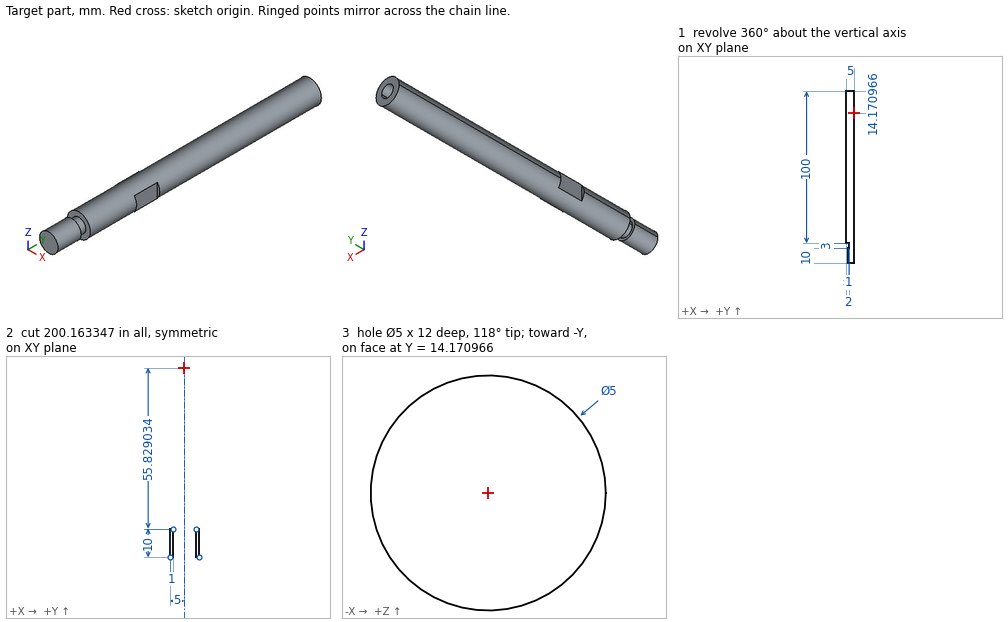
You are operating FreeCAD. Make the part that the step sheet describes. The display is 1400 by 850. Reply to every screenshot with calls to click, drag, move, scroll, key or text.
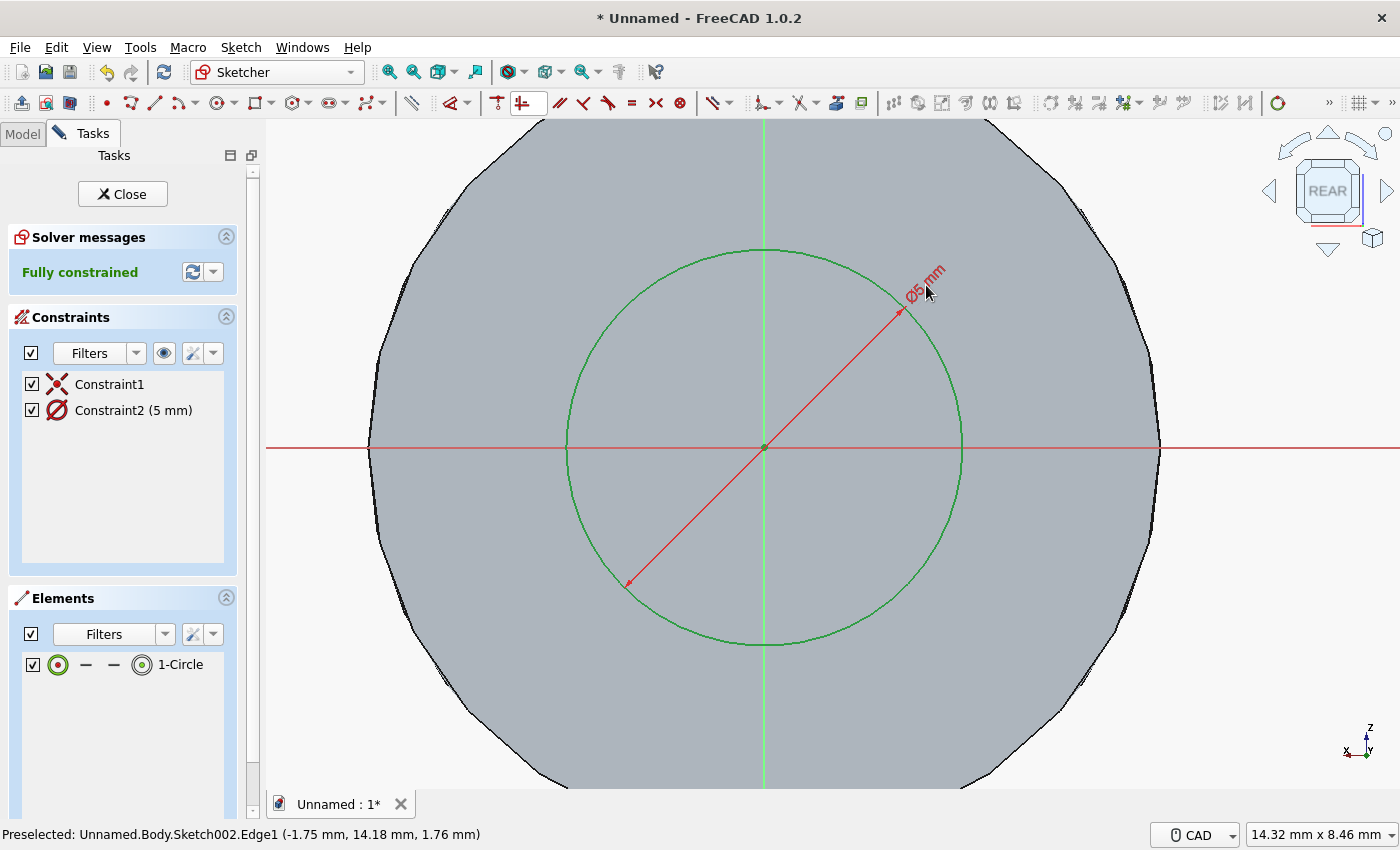
click(123, 194)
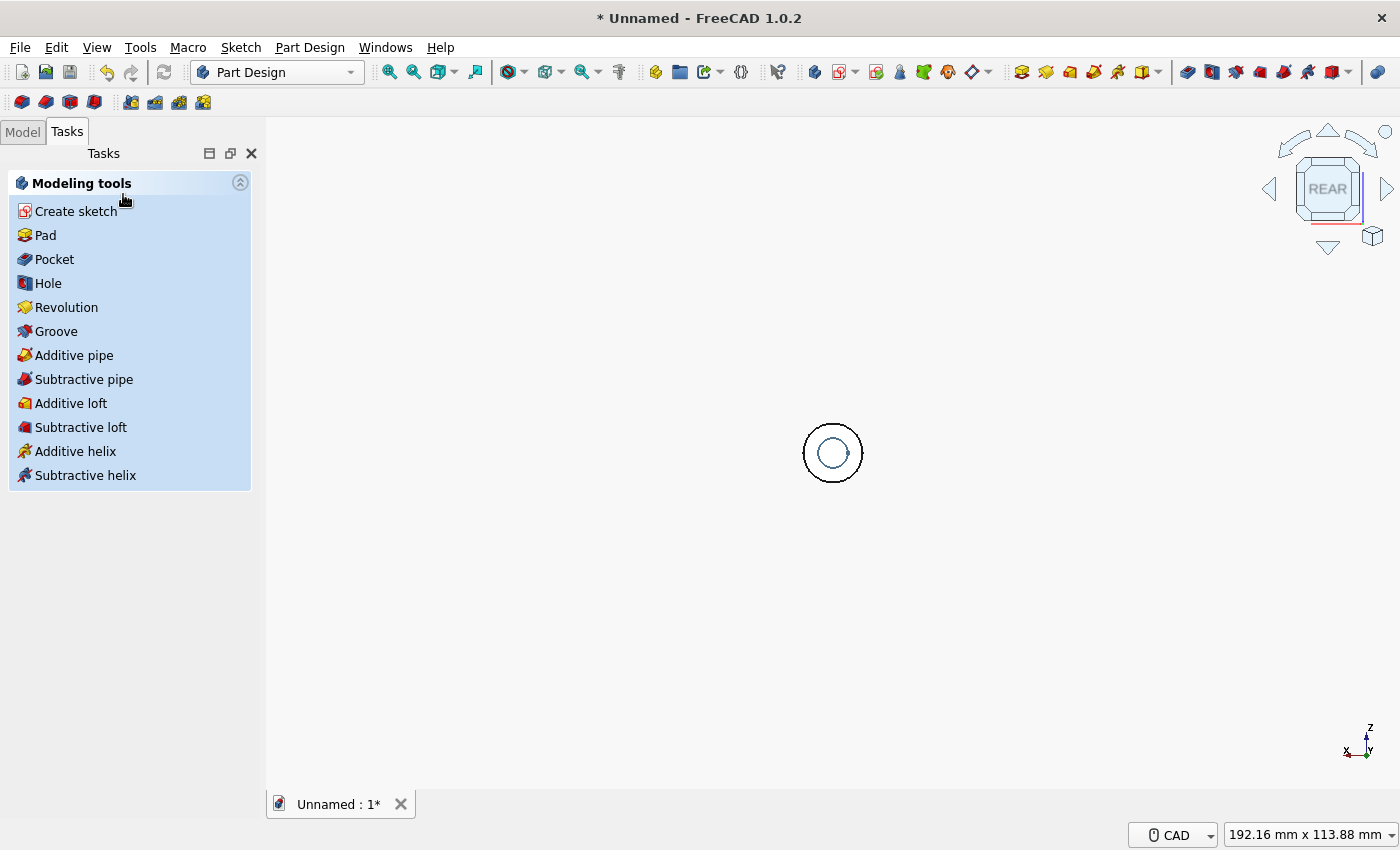
click(1212, 72)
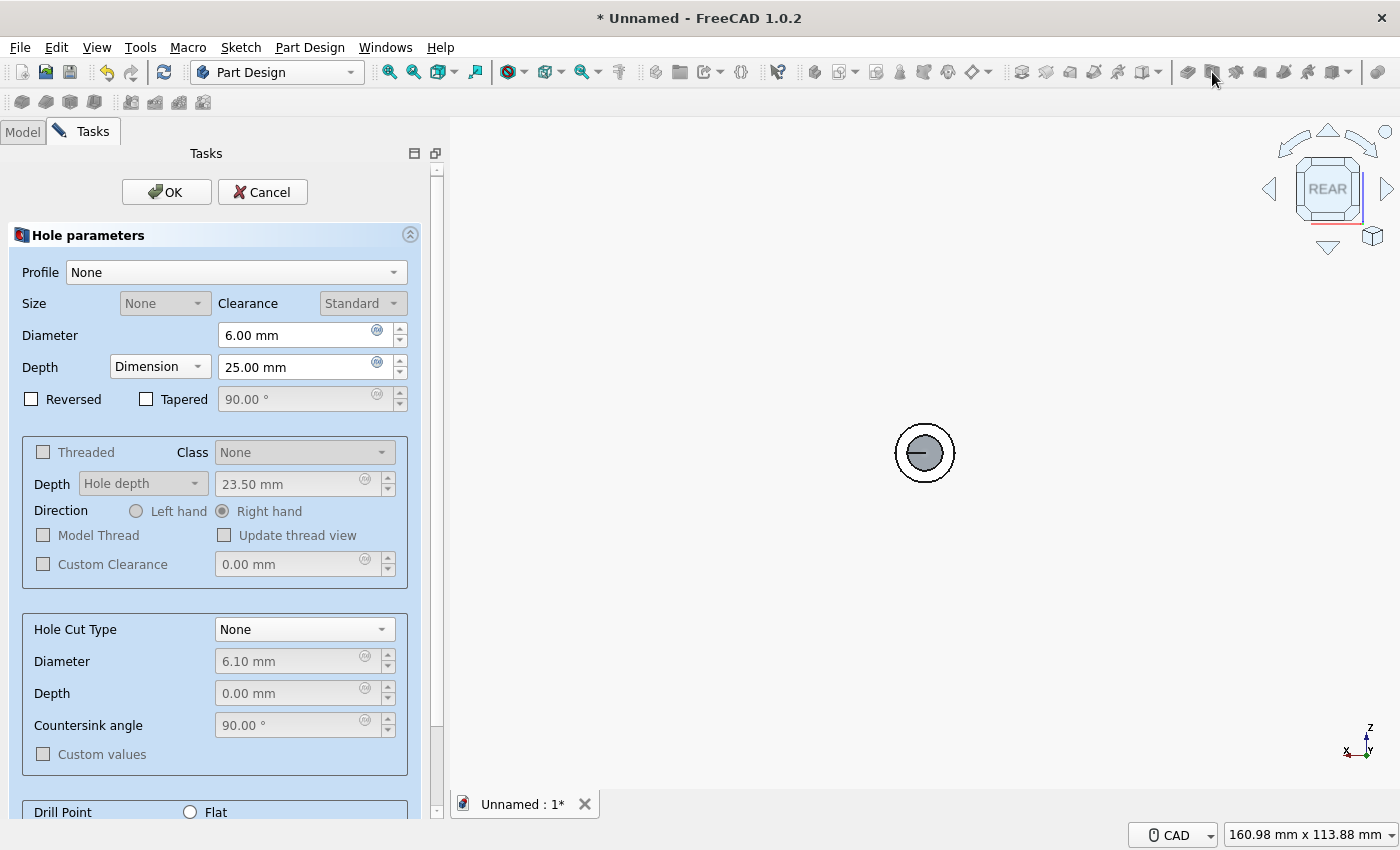
triple_click(305, 335)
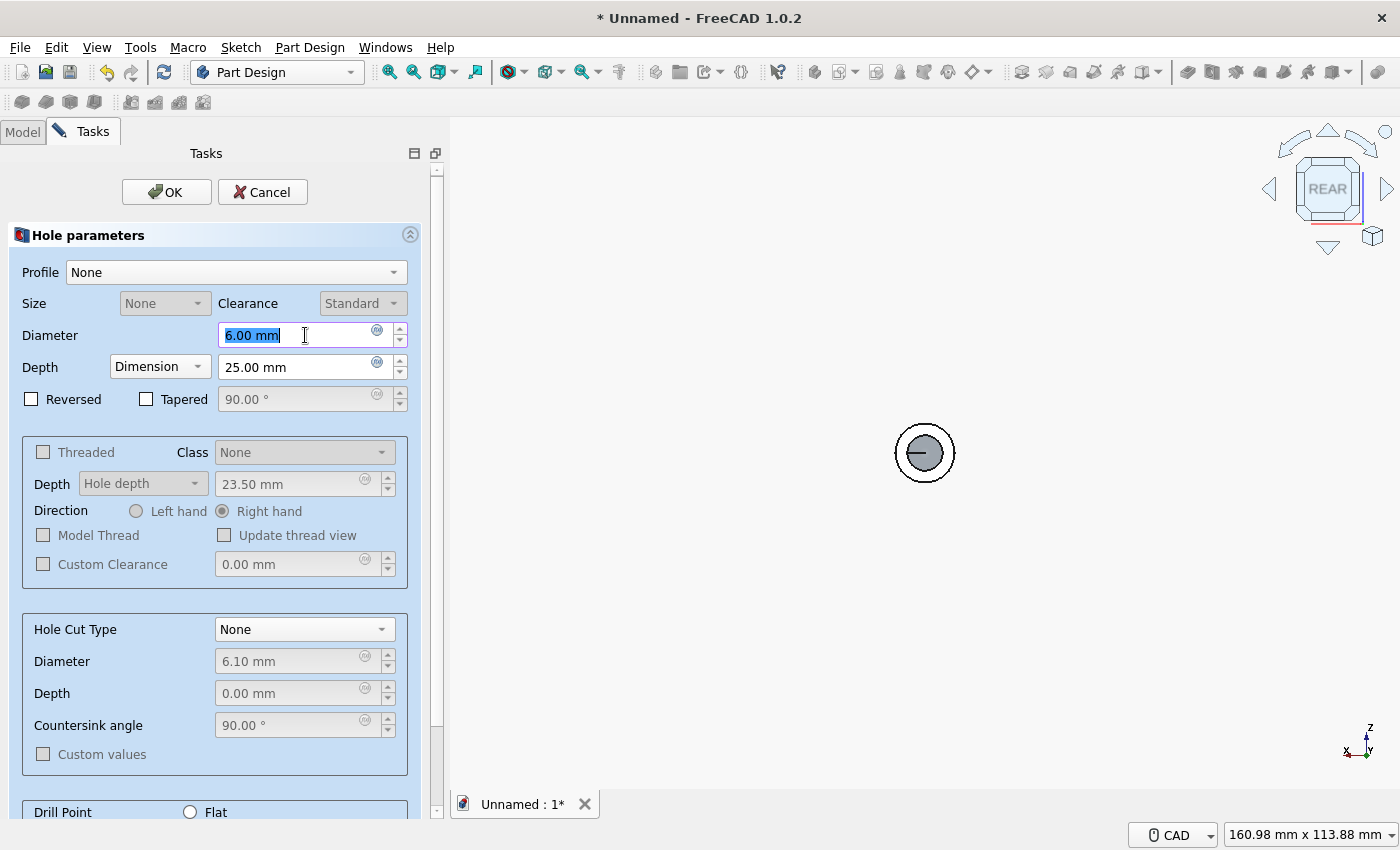
text(5)
key(Tab)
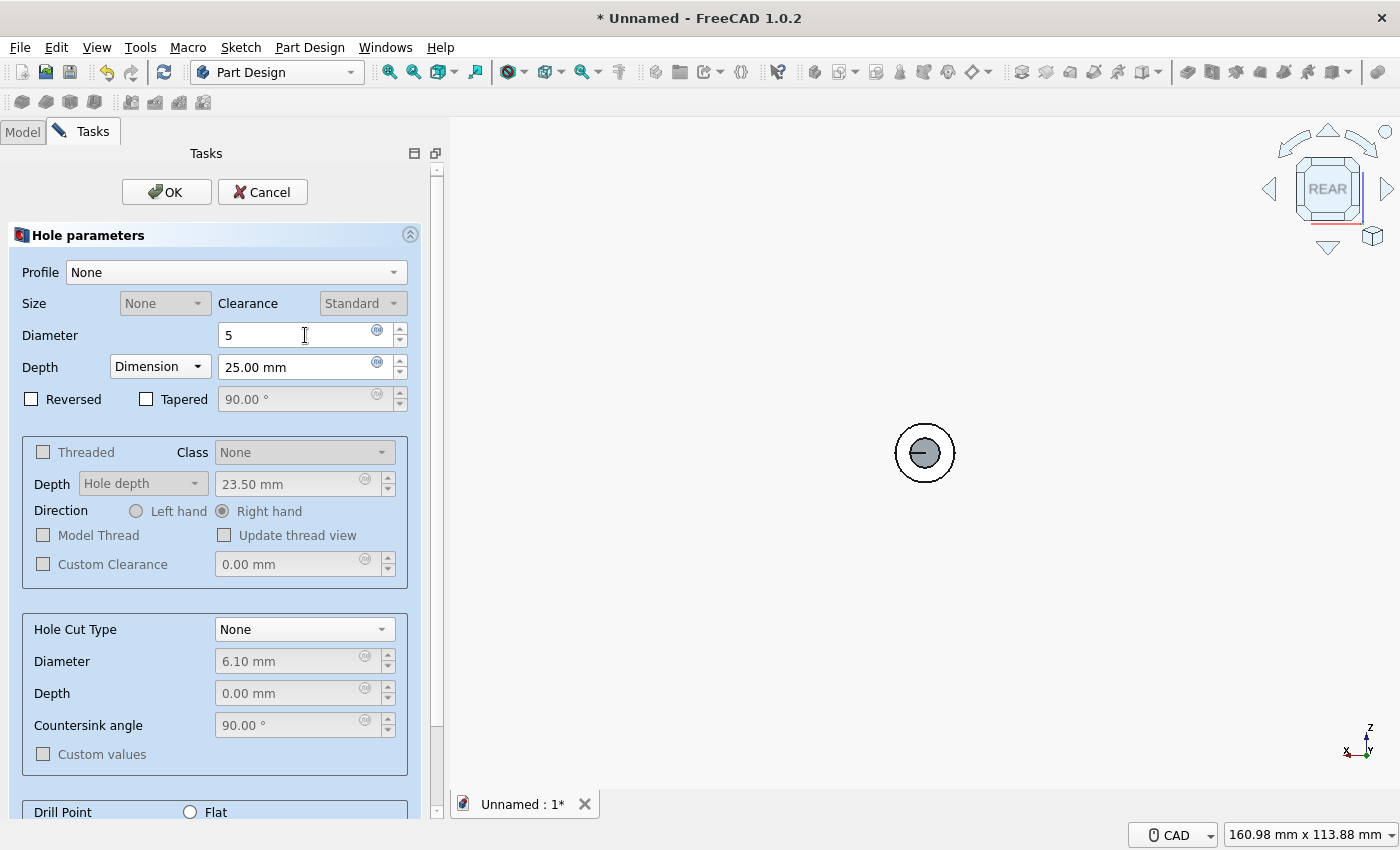
triple_click(305, 367)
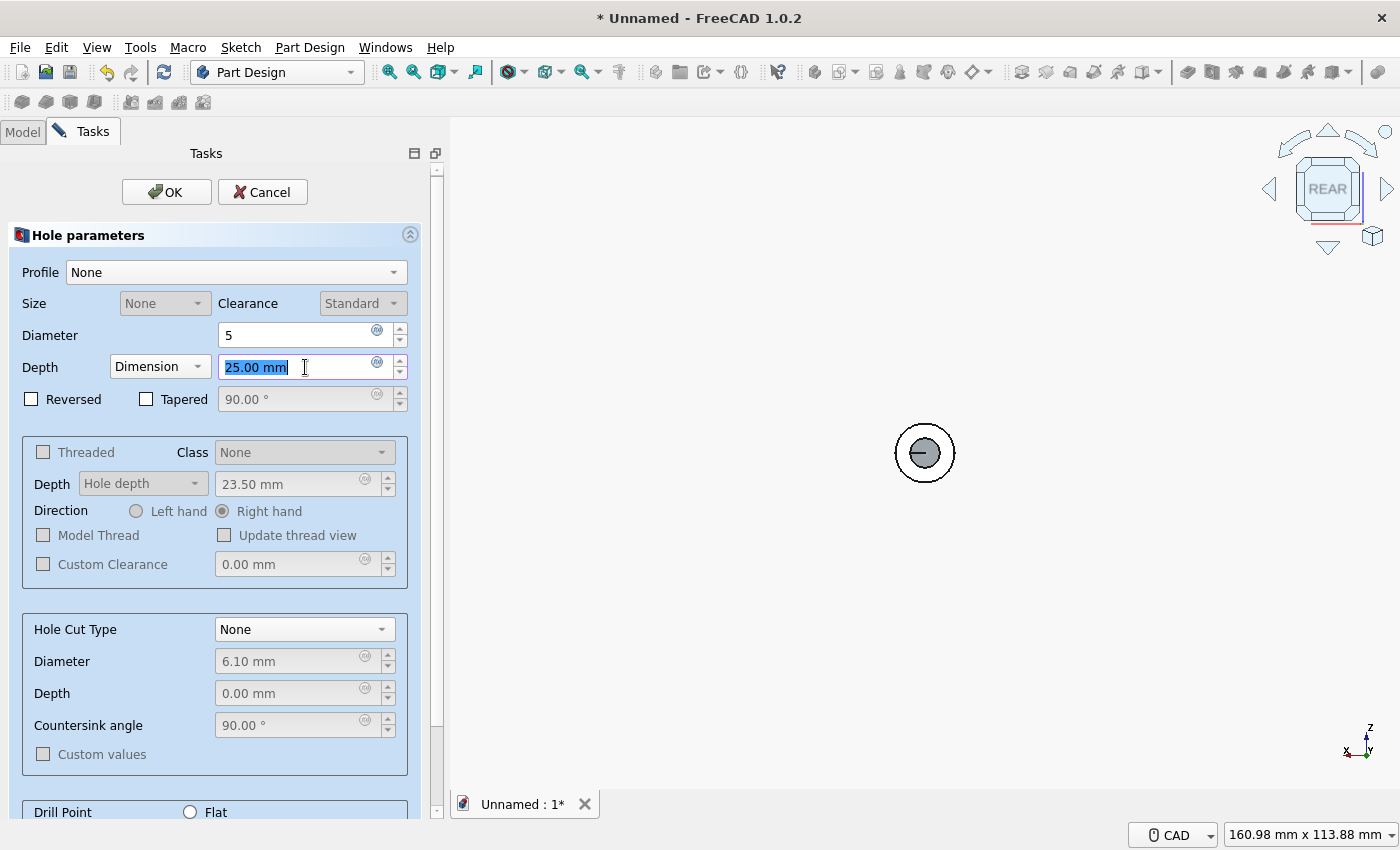
text(12)
key(Tab)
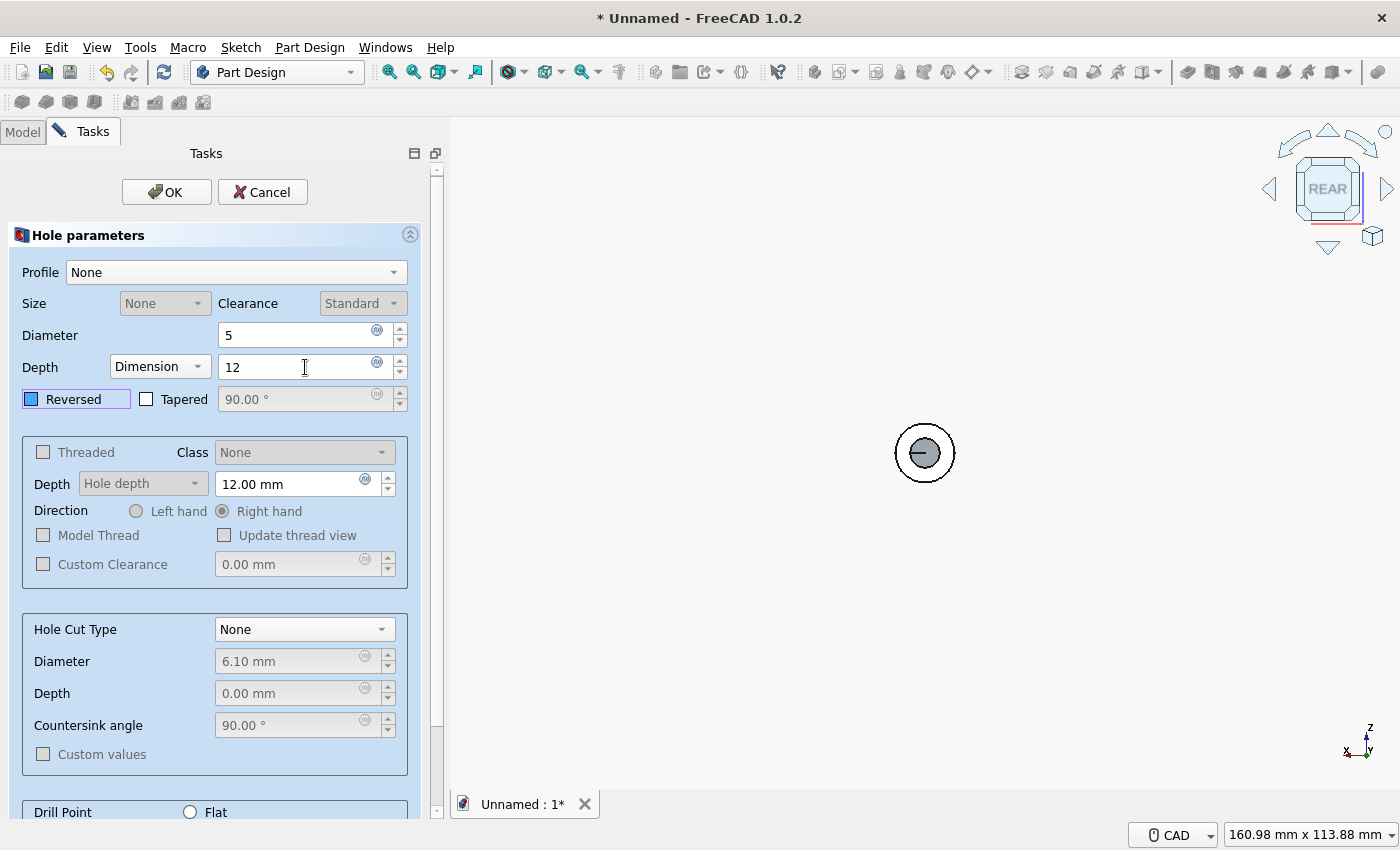
click(167, 192)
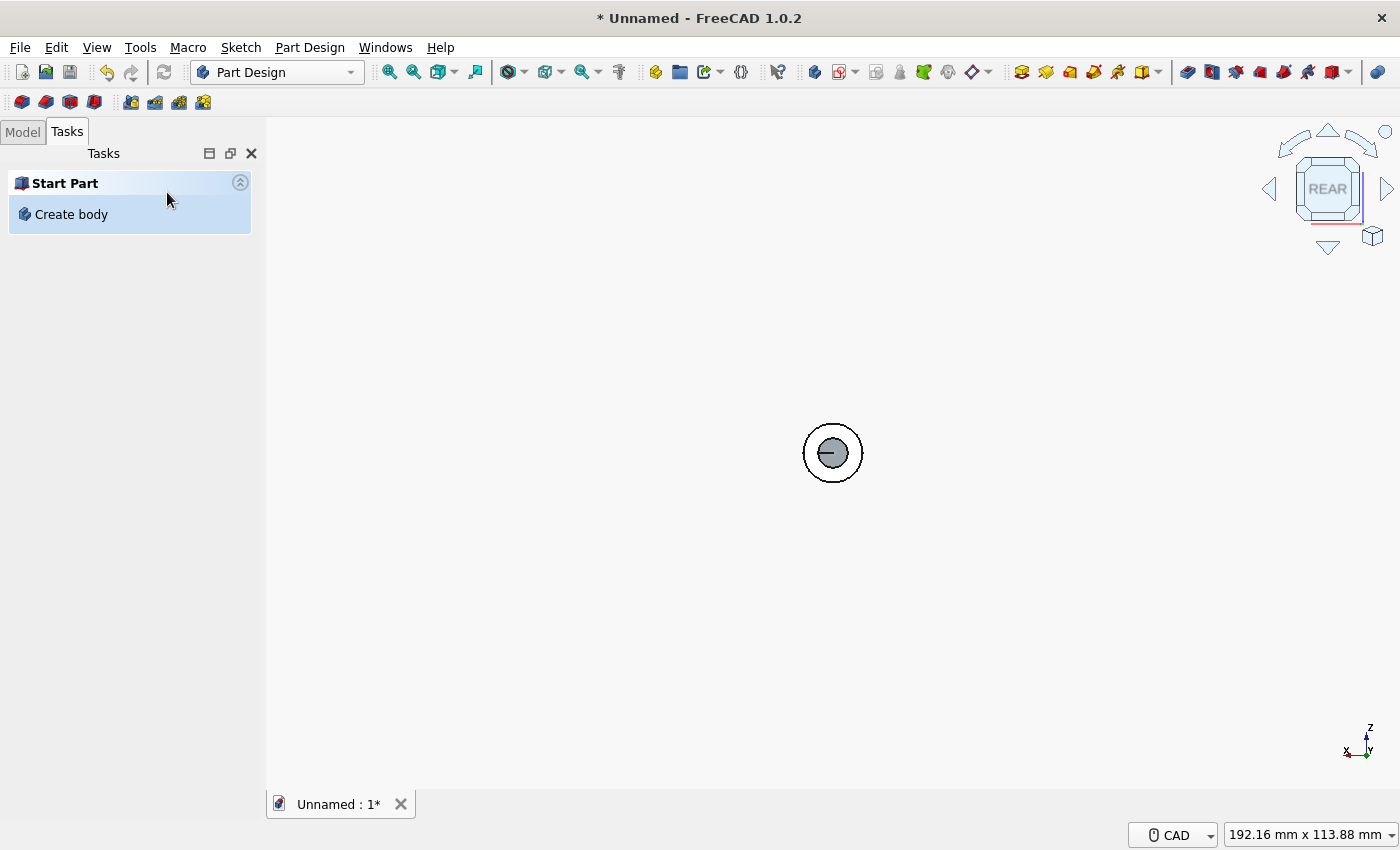
key(0)